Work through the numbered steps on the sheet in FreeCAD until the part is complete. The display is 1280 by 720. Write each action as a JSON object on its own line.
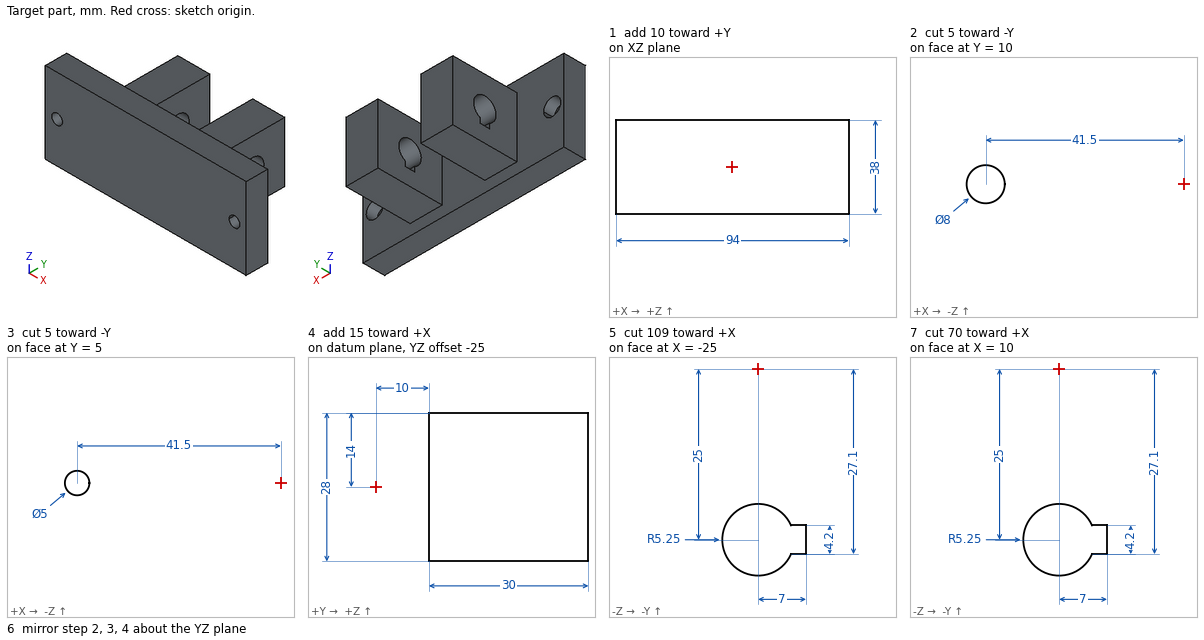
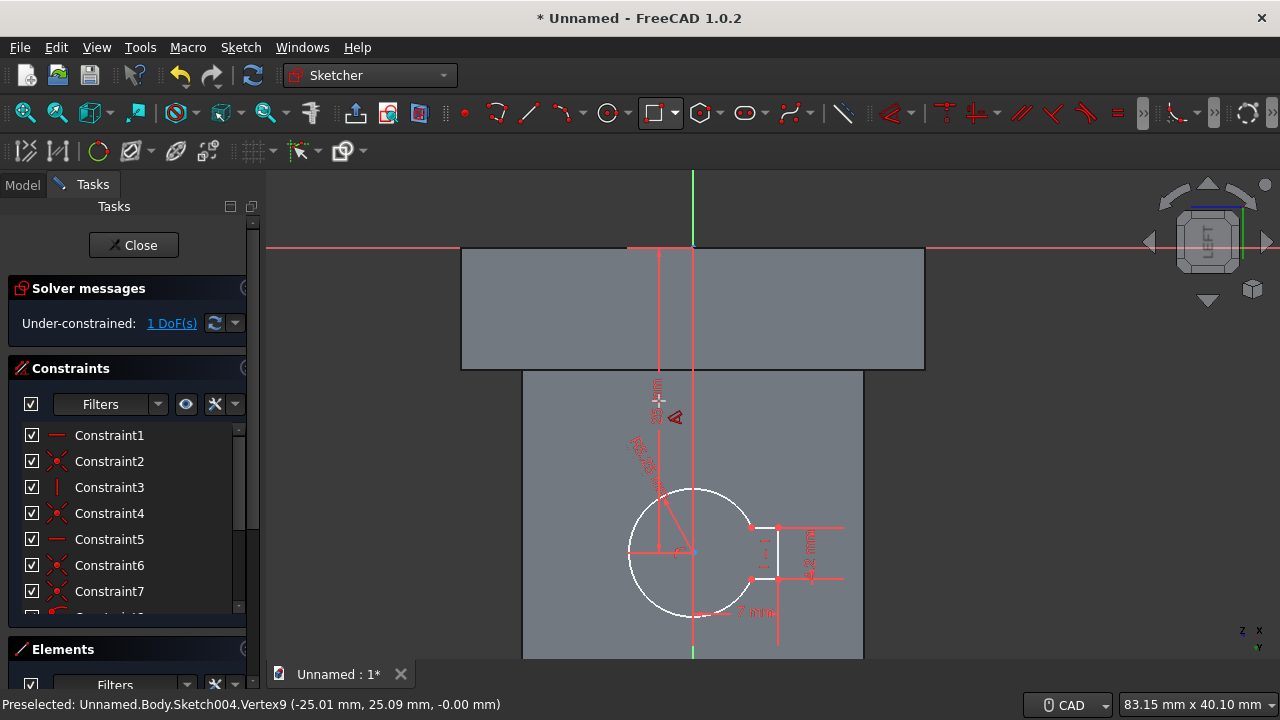
{"action": "left_click", "coordinate": [751, 579]}
{"action": "left_click", "coordinate": [785, 414]}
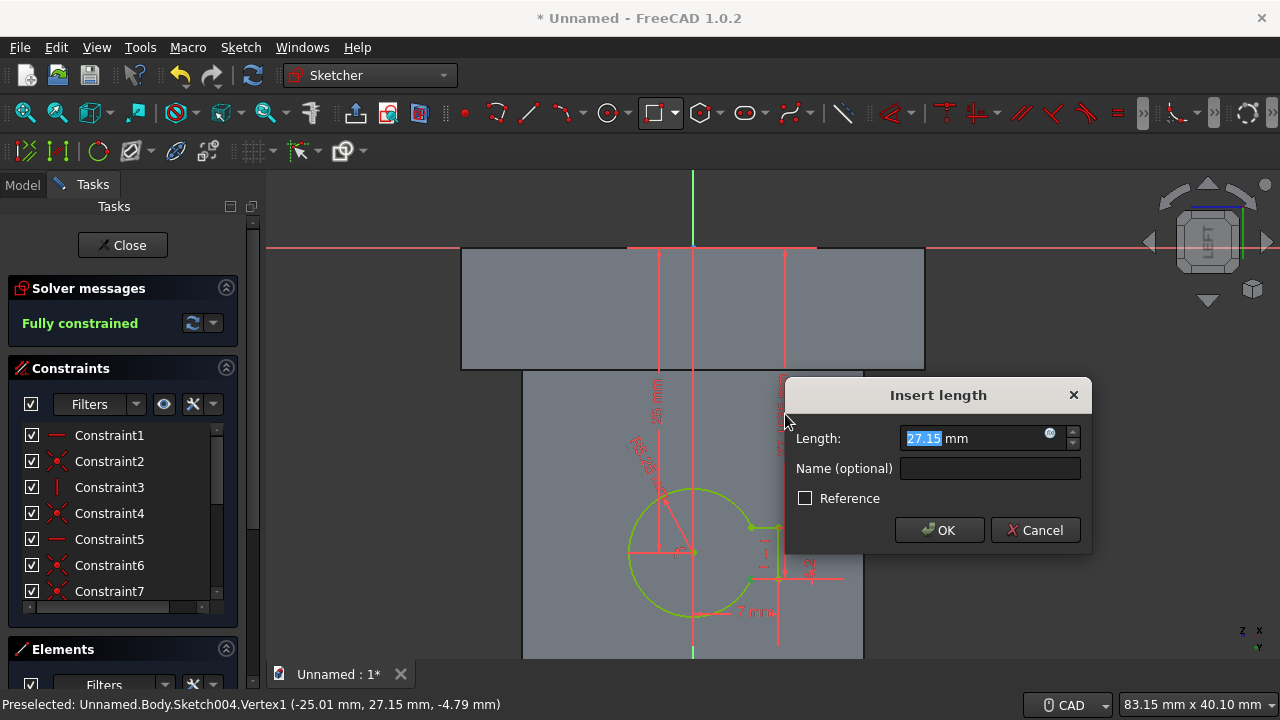
{"action": "type", "text": "27.1"}
{"action": "key", "text": "Return"}
{"action": "key", "text": "Escape"}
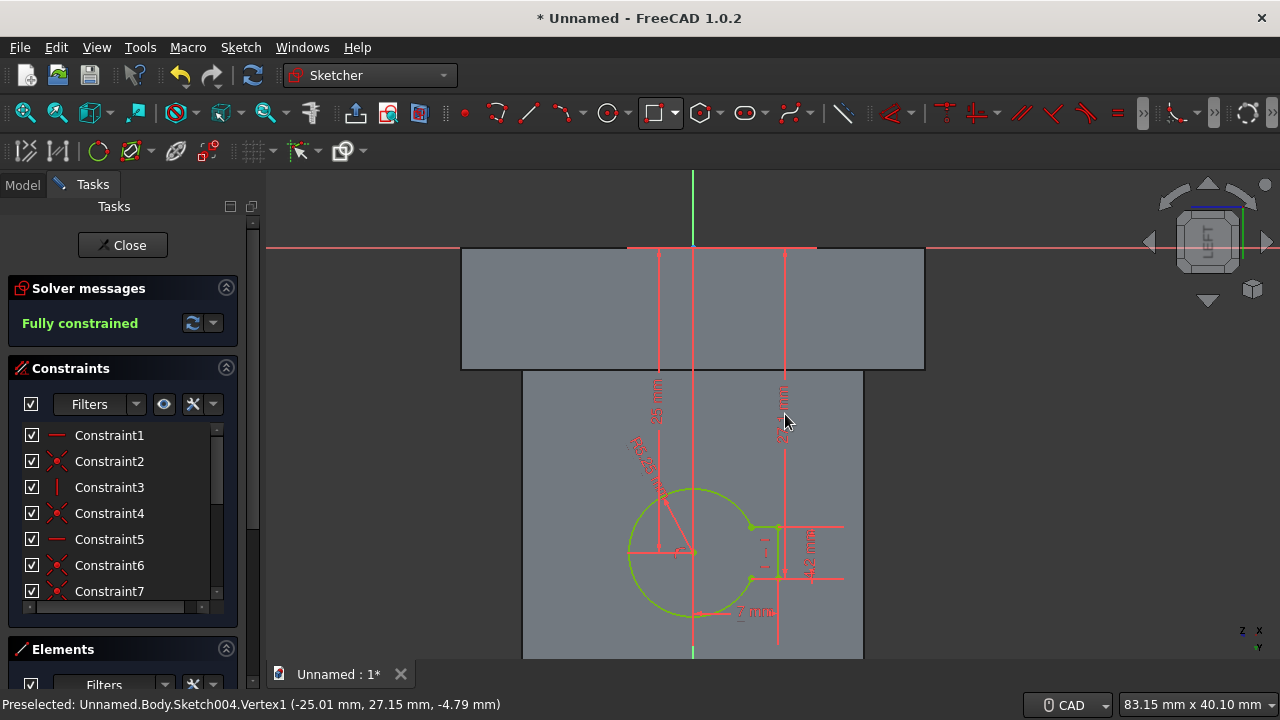
{"action": "left_click", "coordinate": [123, 245]}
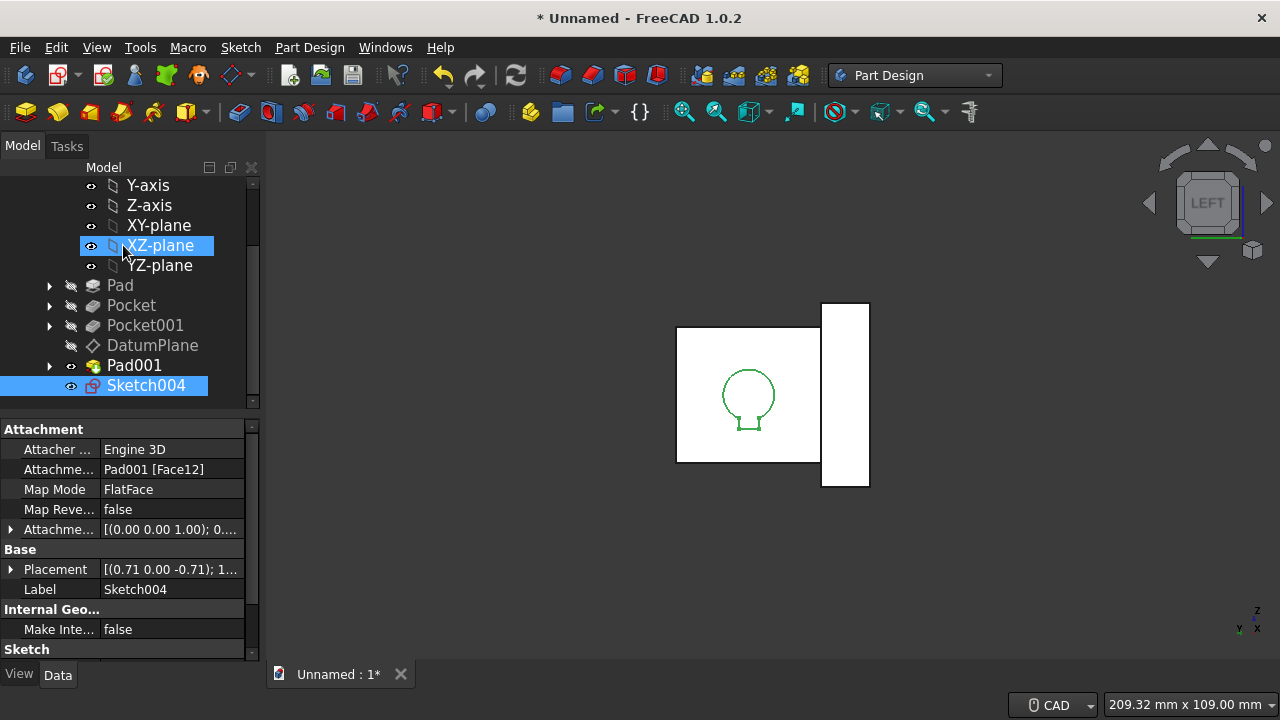
{"action": "left_click", "coordinate": [240, 112]}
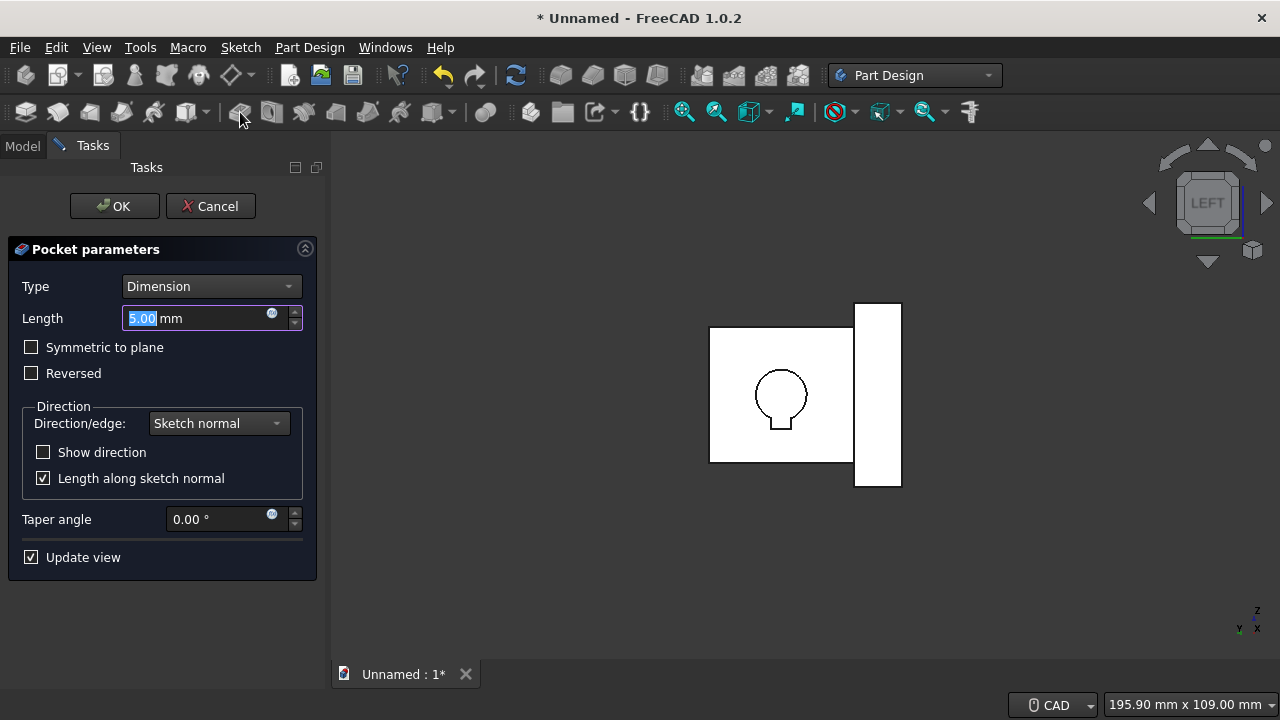
{"action": "type", "text": "109"}
{"action": "key", "text": "Tab"}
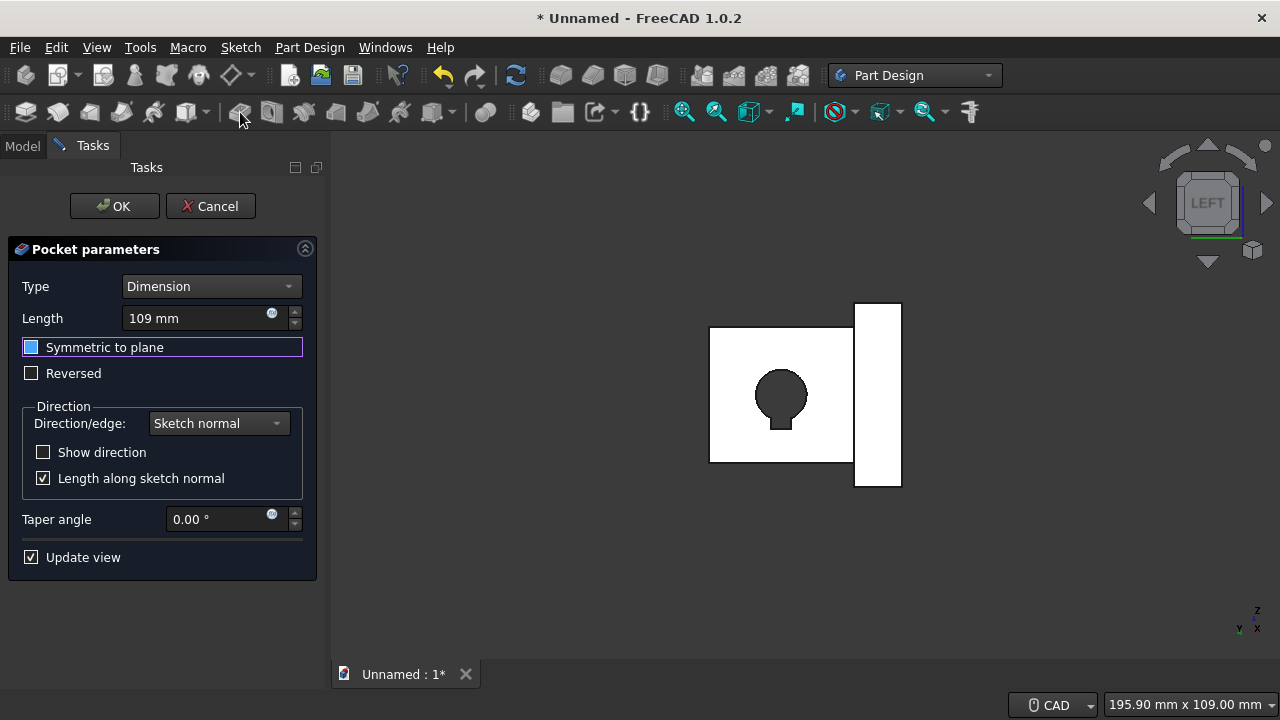
{"action": "left_click", "coordinate": [115, 206]}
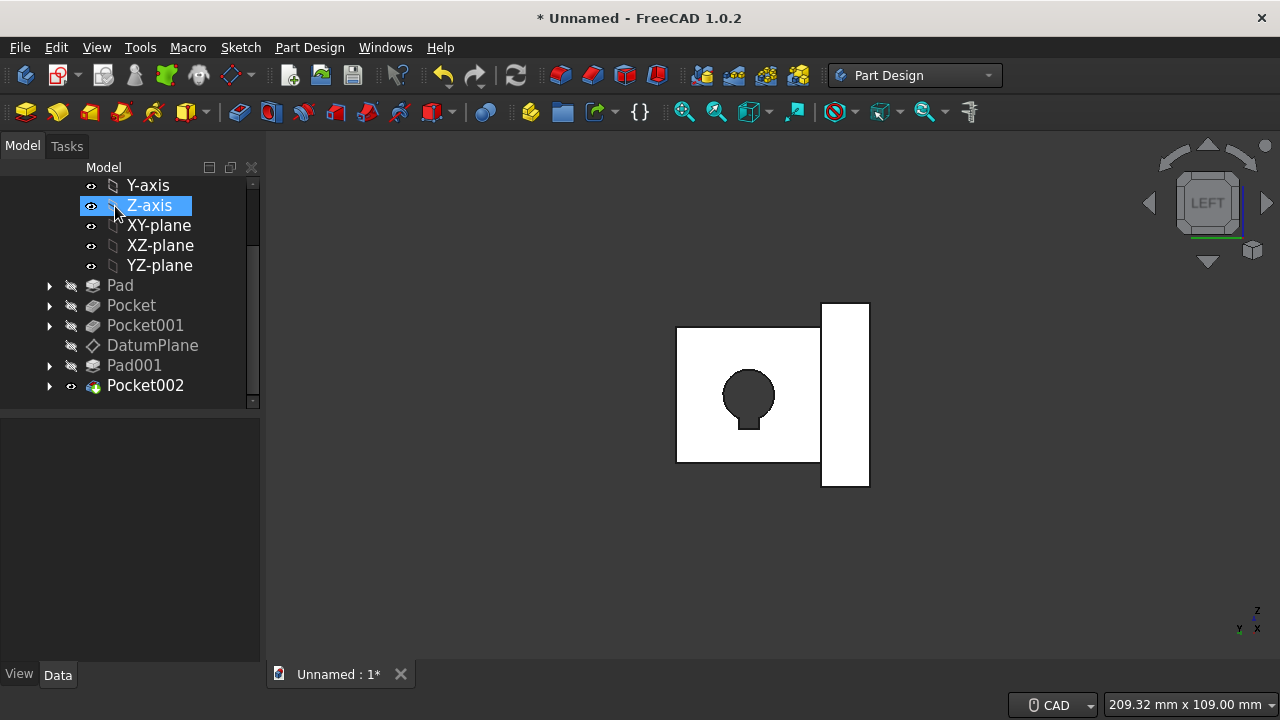
{"action": "left_click", "coordinate": [686, 112]}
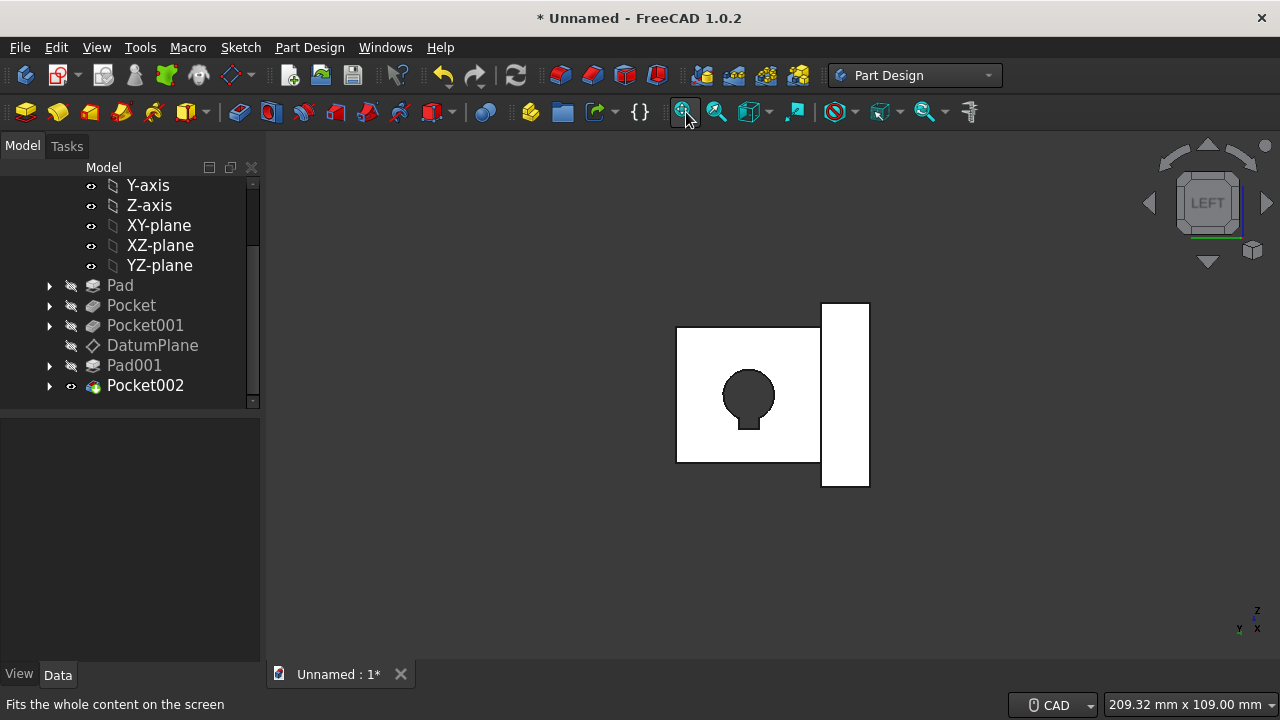
{"action": "left_click", "coordinate": [116, 306]}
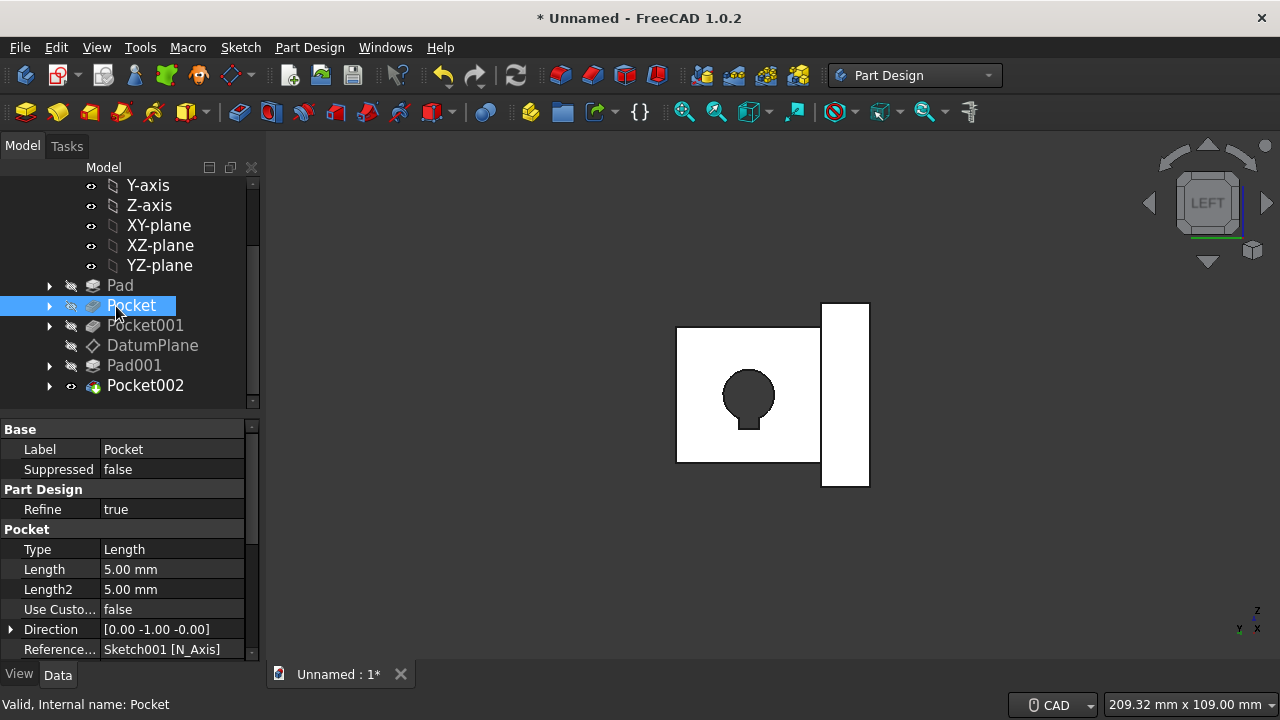
{"action": "left_click", "coordinate": [116, 326], "text": "ctrl"}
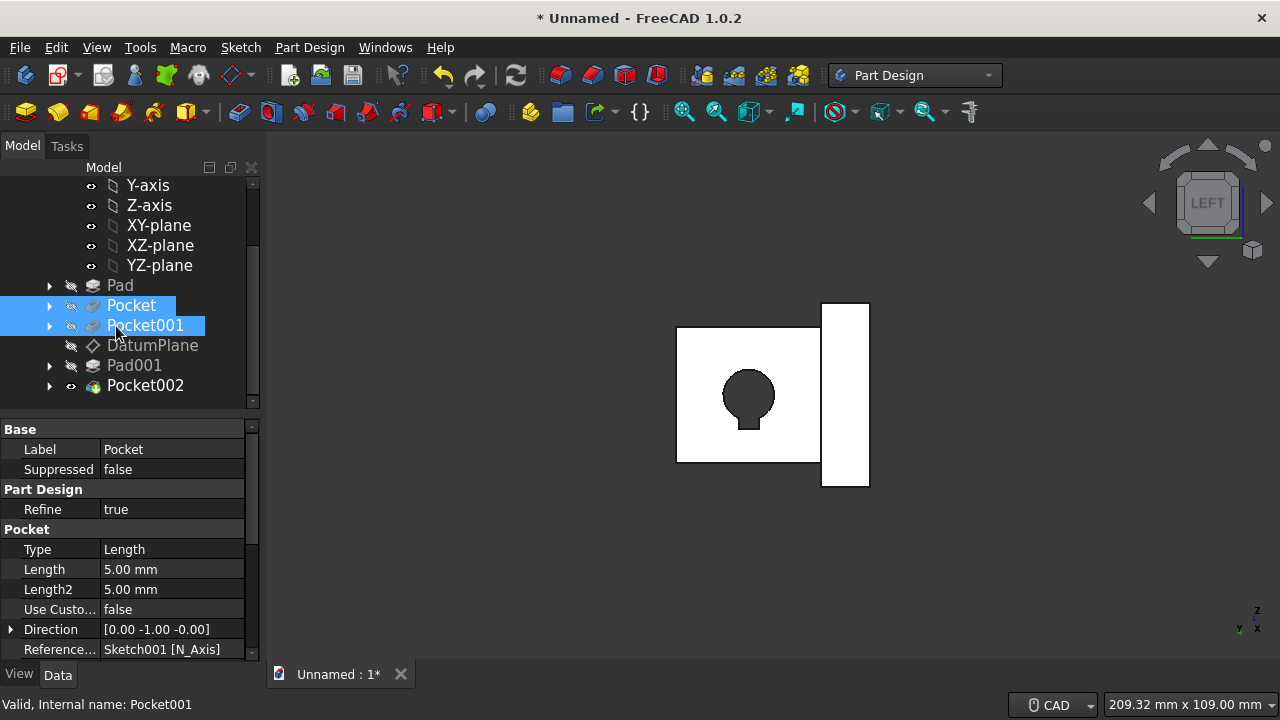
{"action": "left_click", "coordinate": [116, 366], "text": "ctrl"}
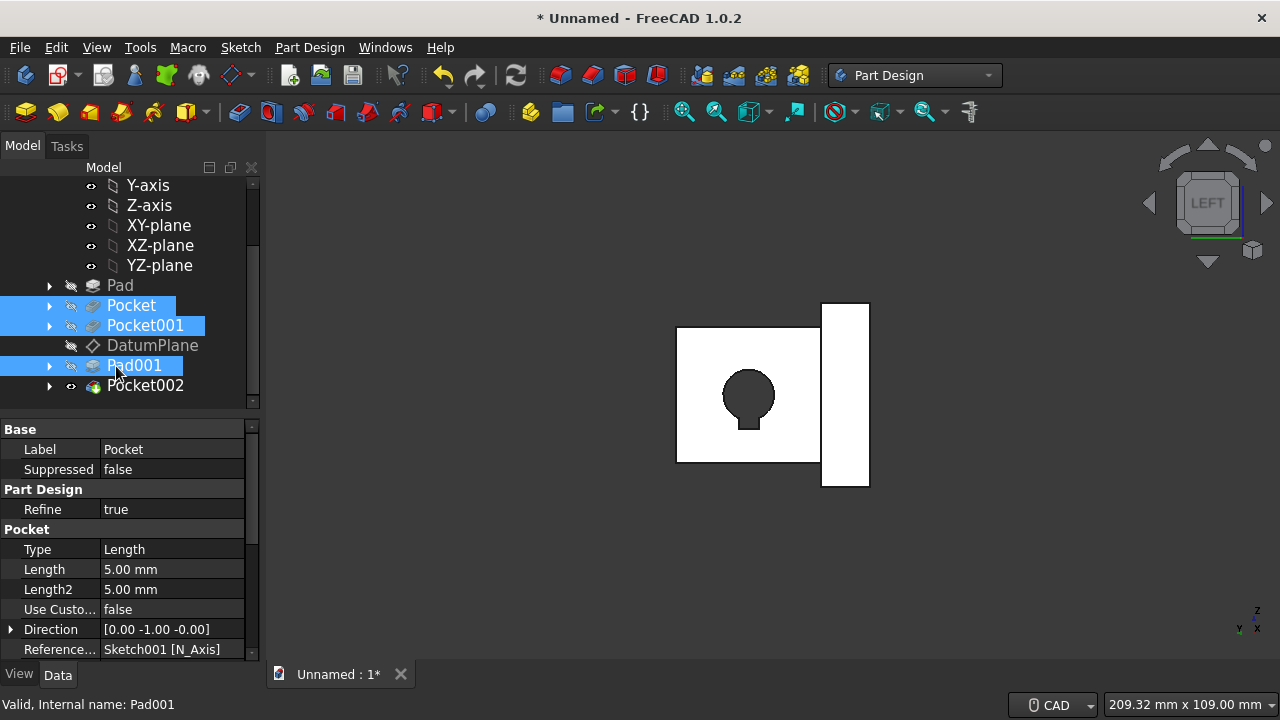
{"action": "left_click", "coordinate": [702, 76]}